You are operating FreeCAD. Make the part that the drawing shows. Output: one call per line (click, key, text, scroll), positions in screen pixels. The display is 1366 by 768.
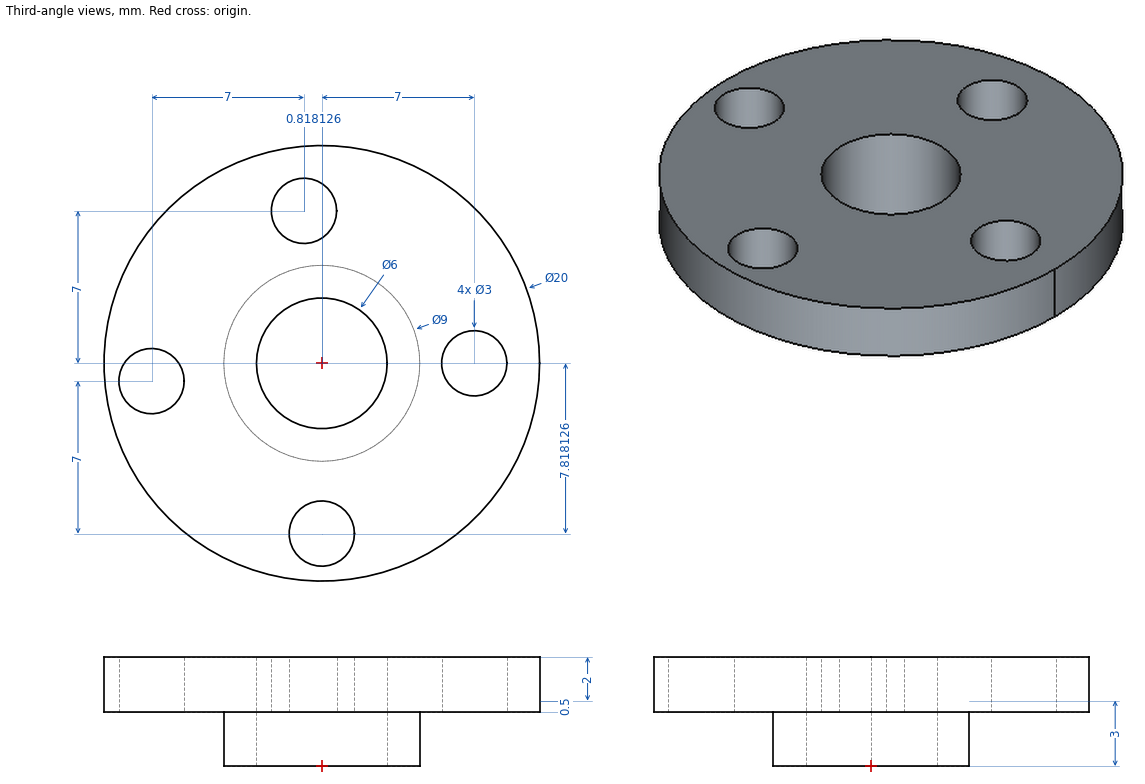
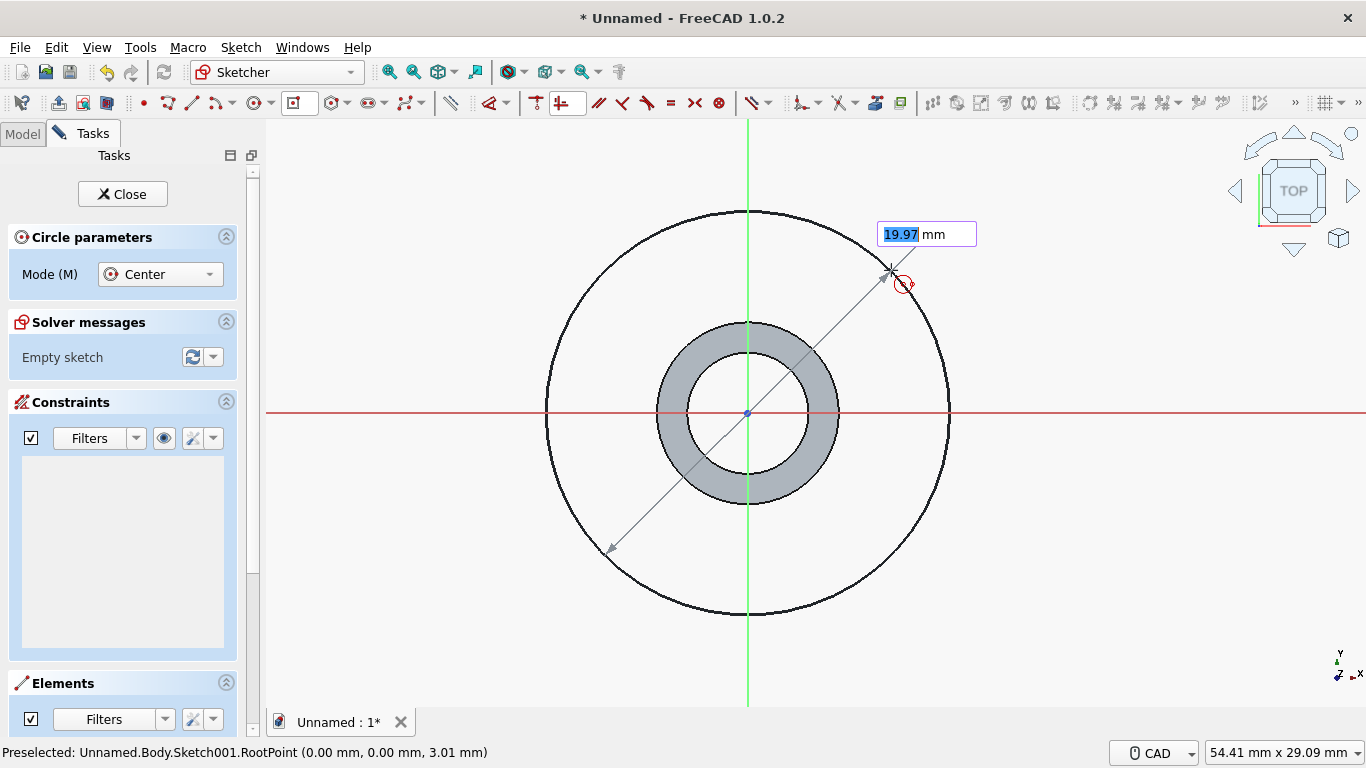
text(20)
key(Return)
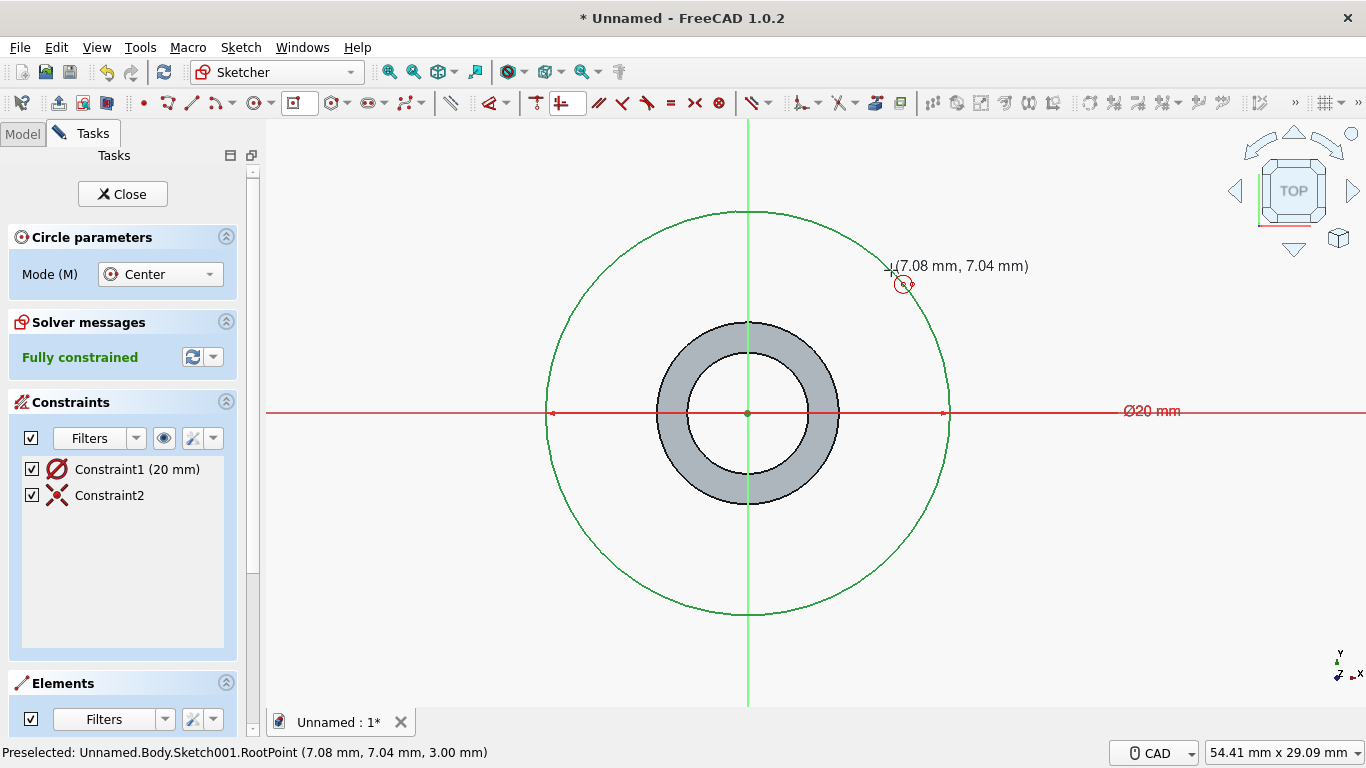
click(748, 413)
move(791, 370)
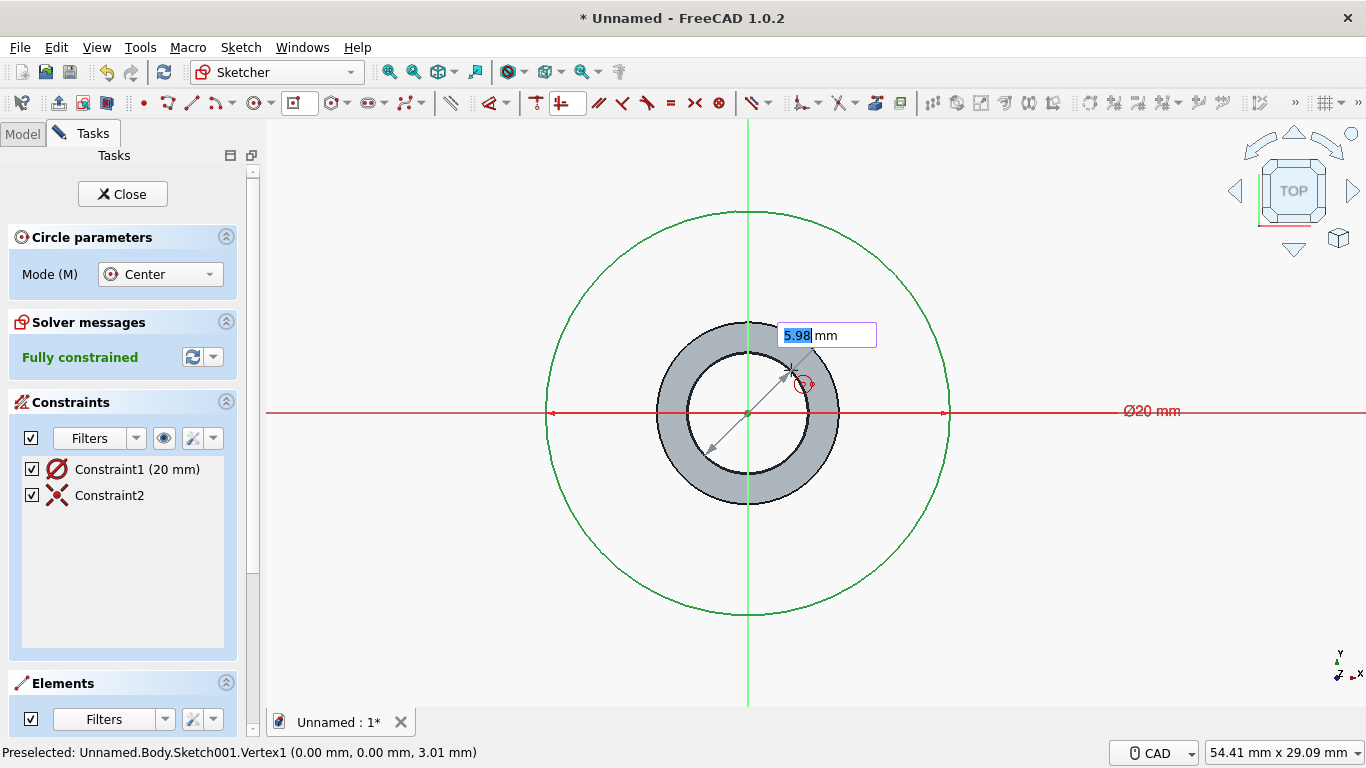
text(6)
key(Return)
key(Escape)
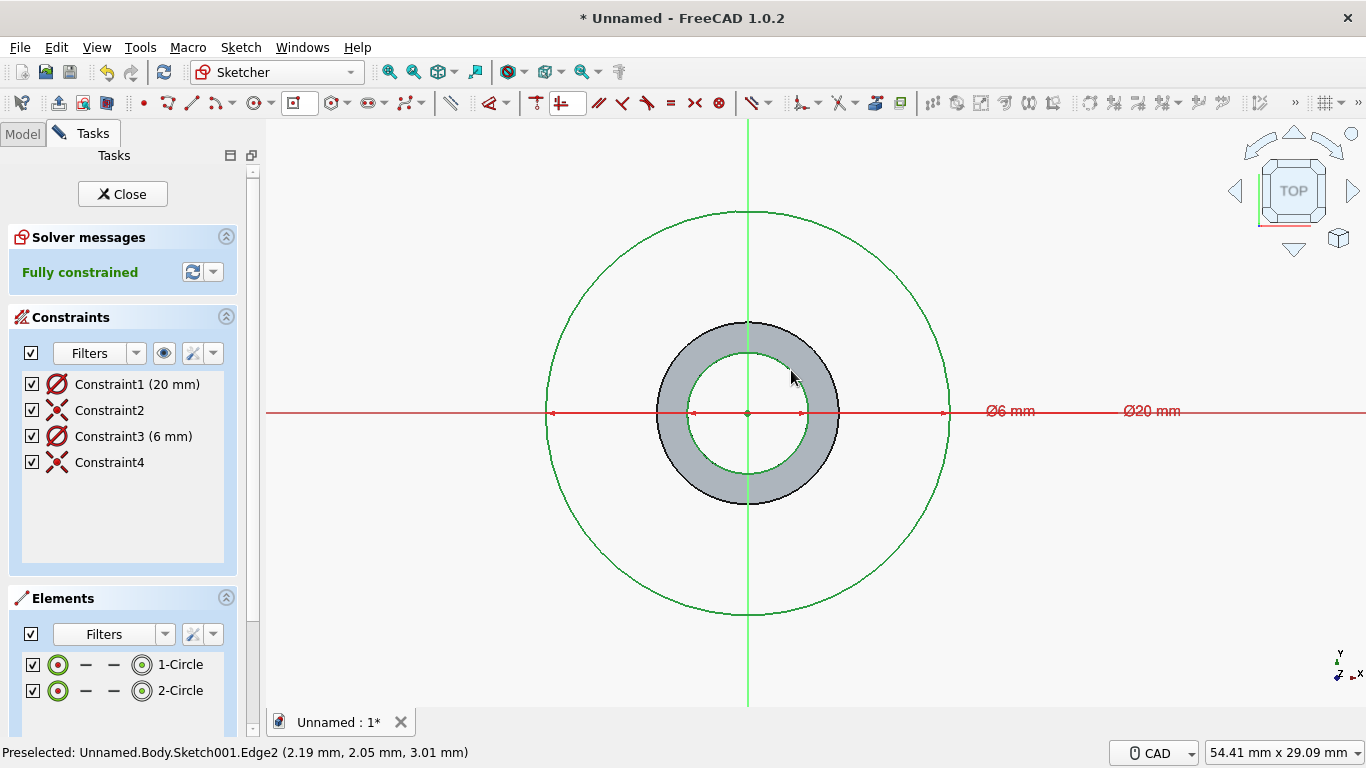
click(123, 194)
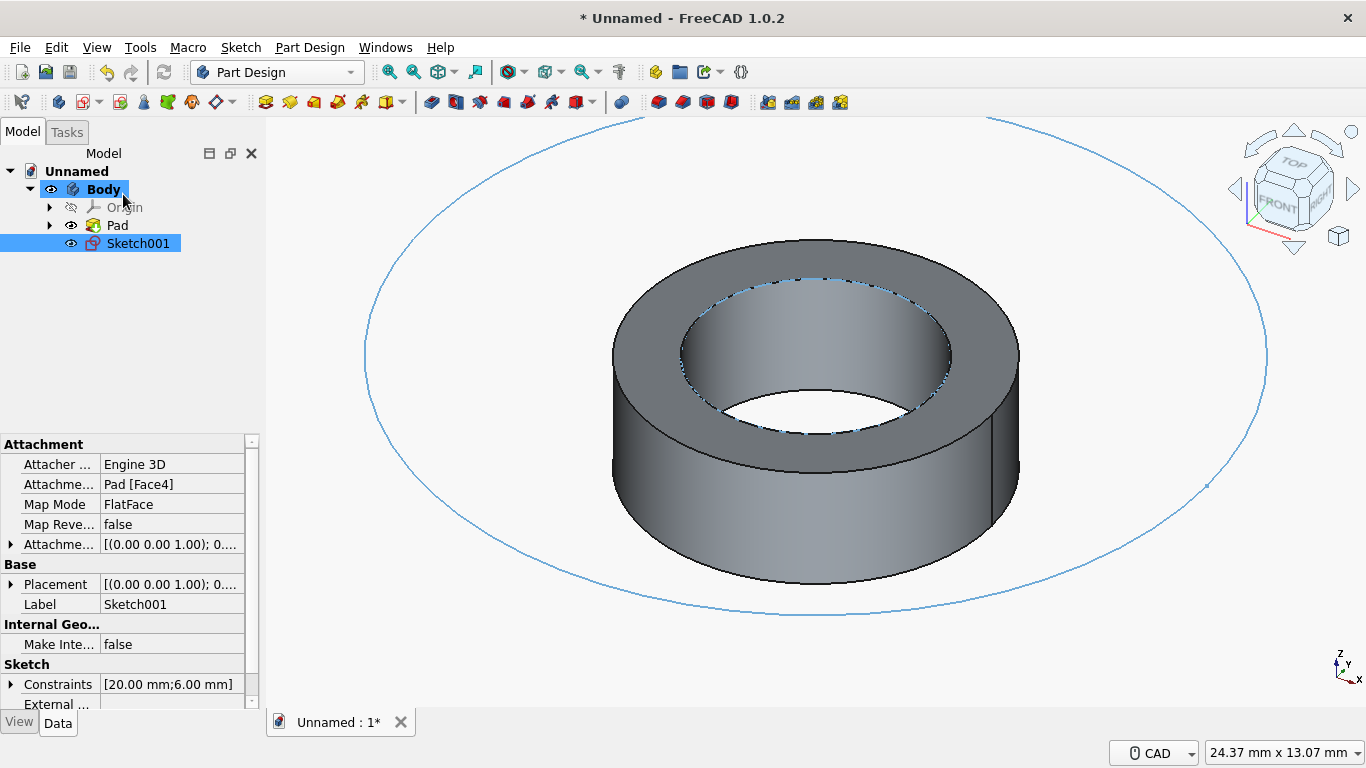
click(266, 102)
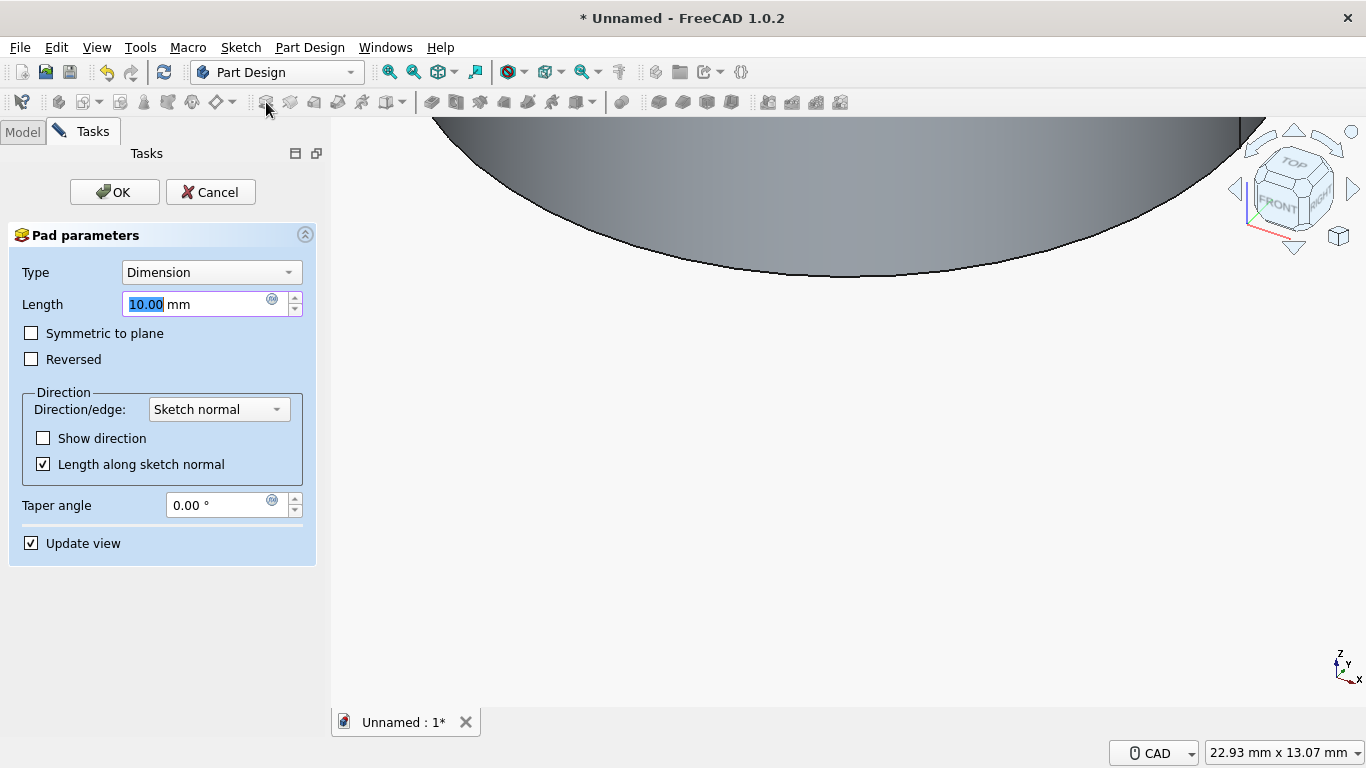
click(212, 272)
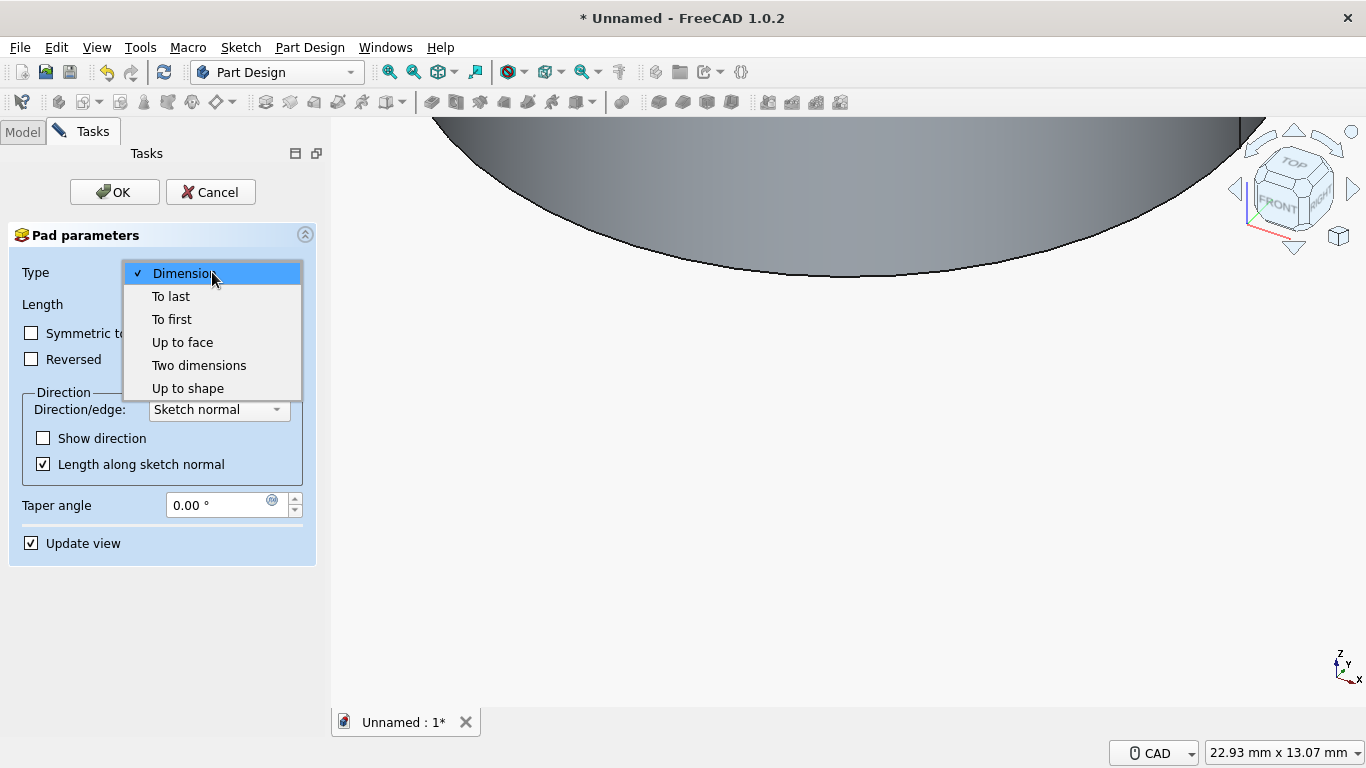
click(212, 366)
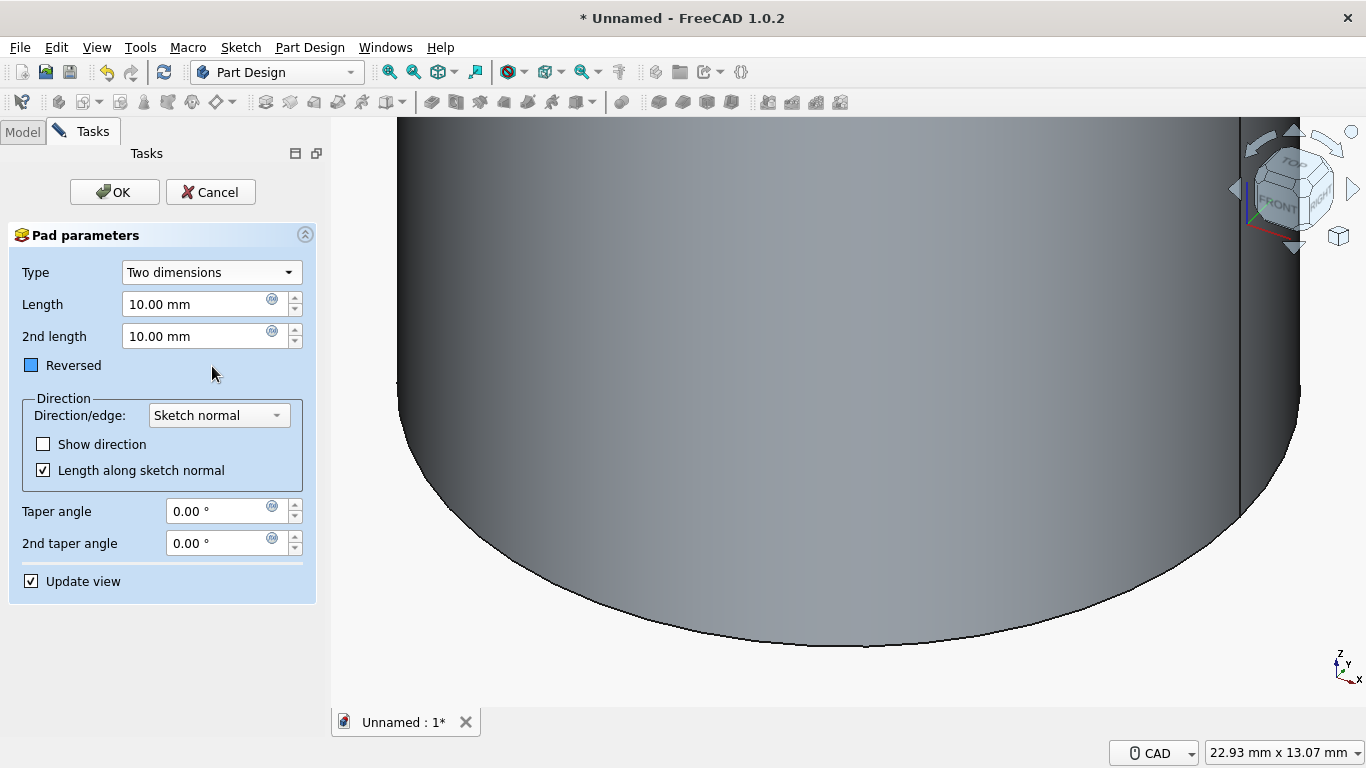
triple_click(204, 304)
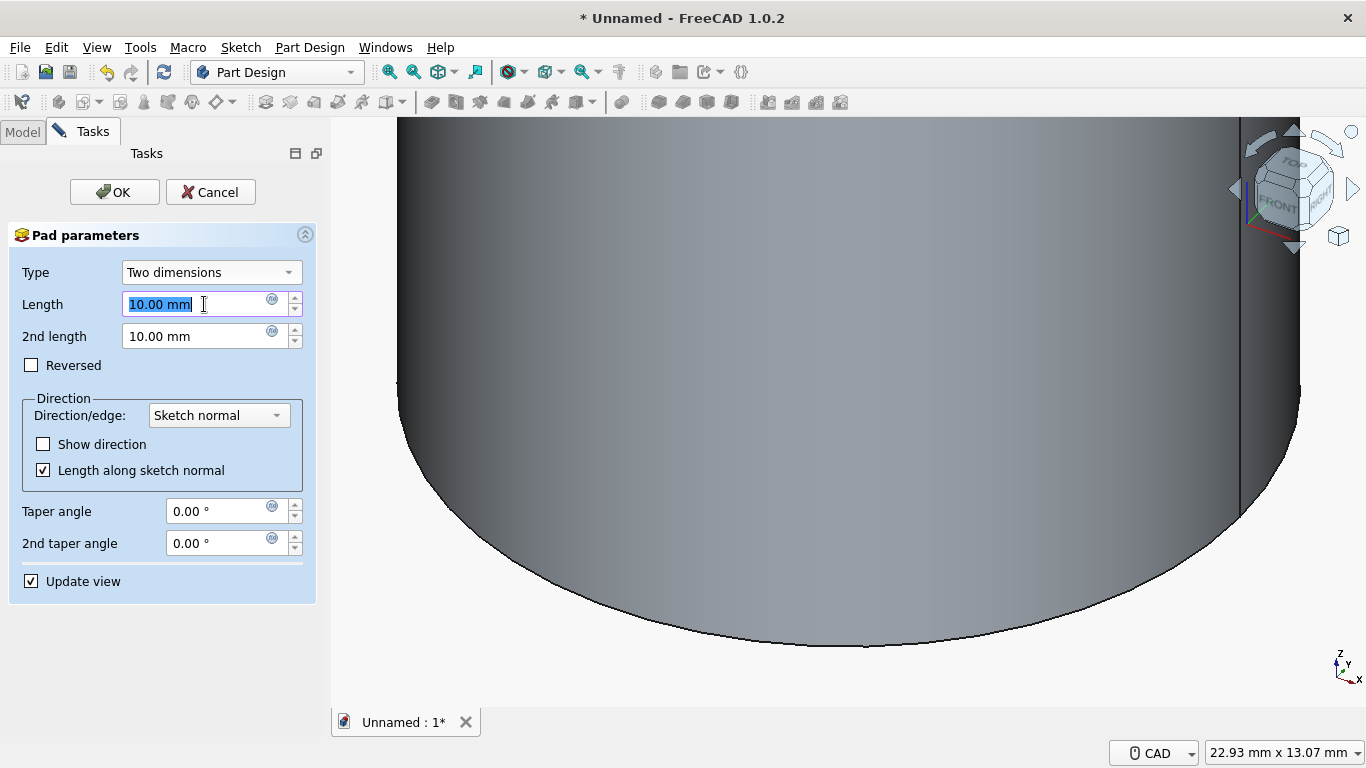
text(2)
key(Tab)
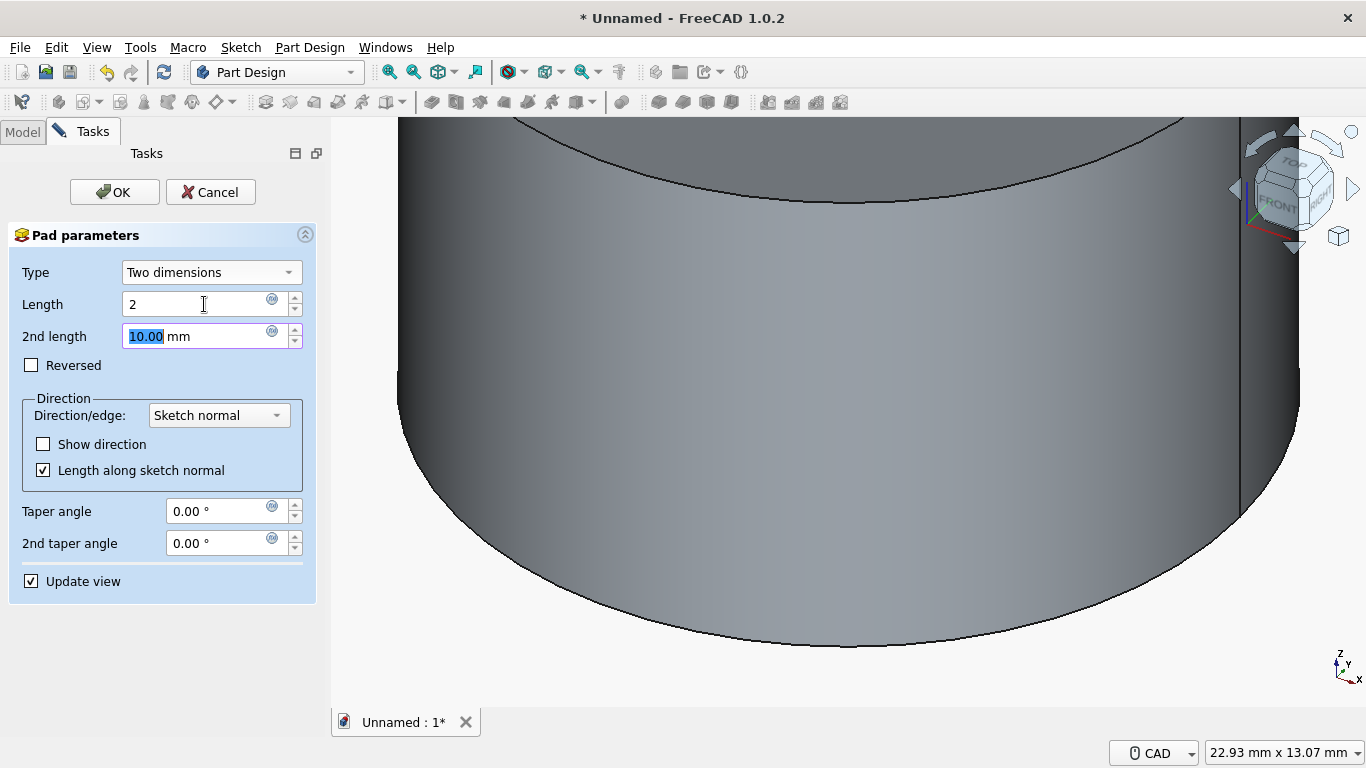
text(0.5)
key(Tab)